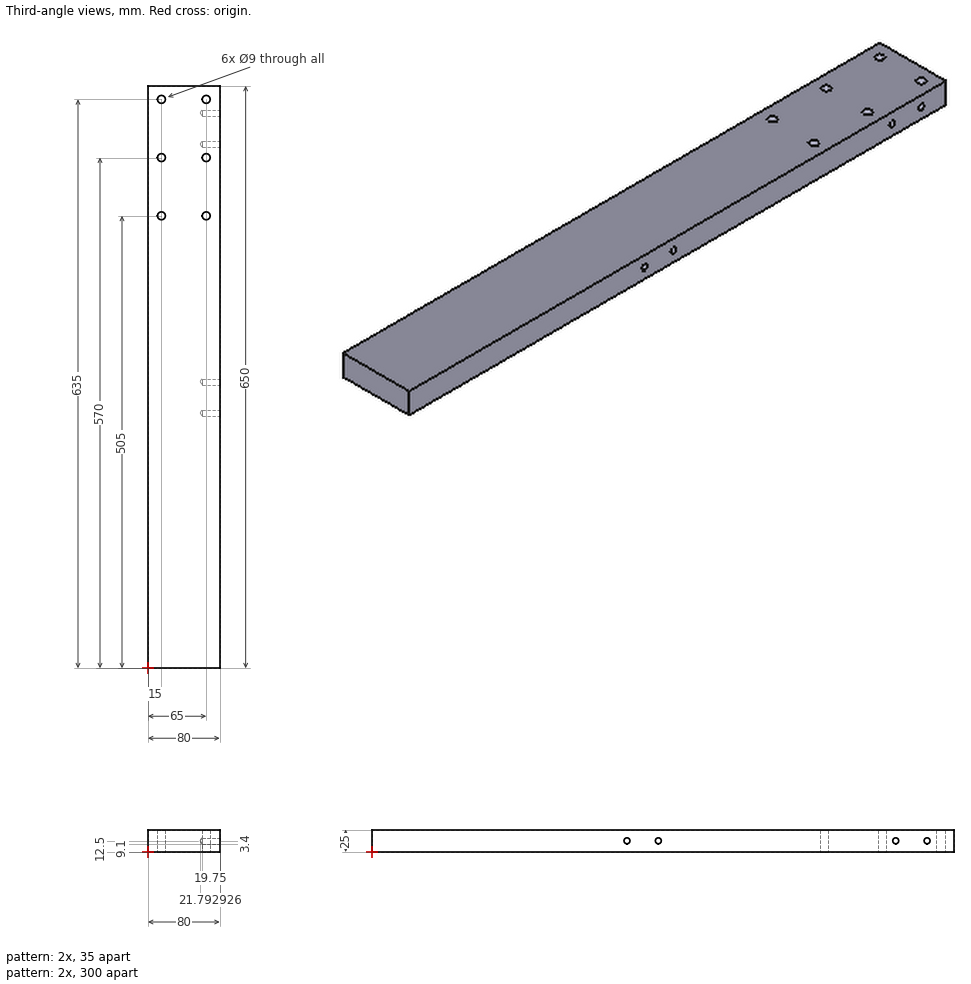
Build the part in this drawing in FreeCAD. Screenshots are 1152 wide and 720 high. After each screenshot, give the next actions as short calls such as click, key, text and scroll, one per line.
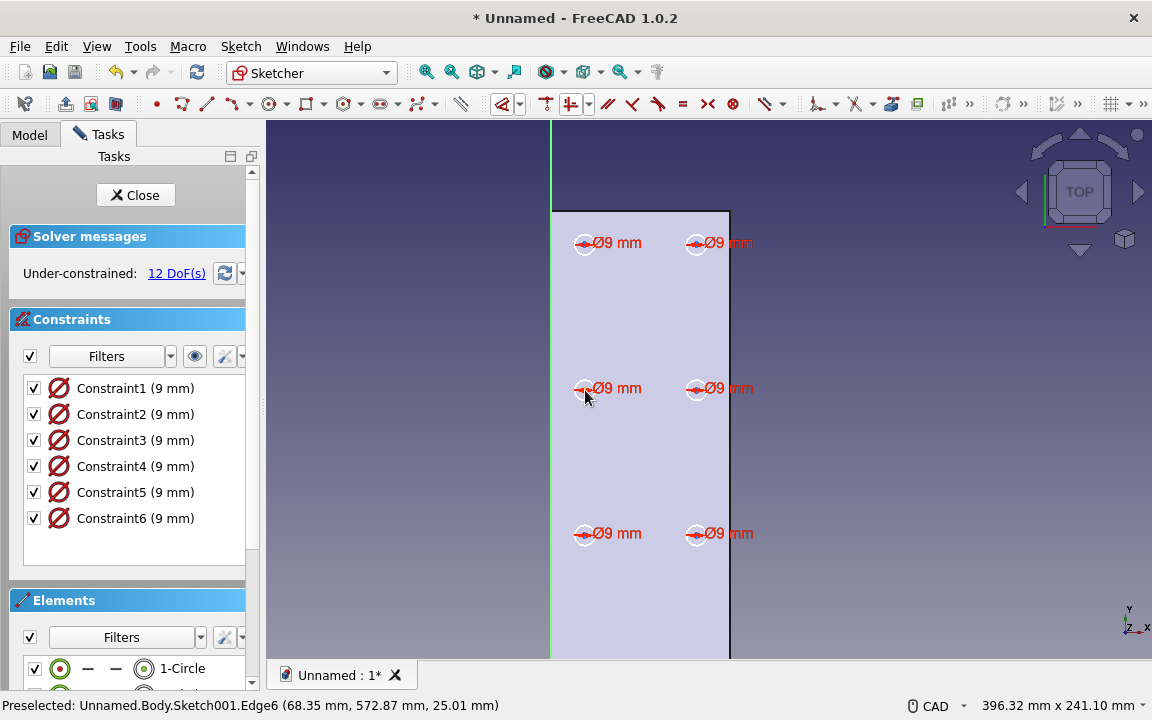
click(585, 245)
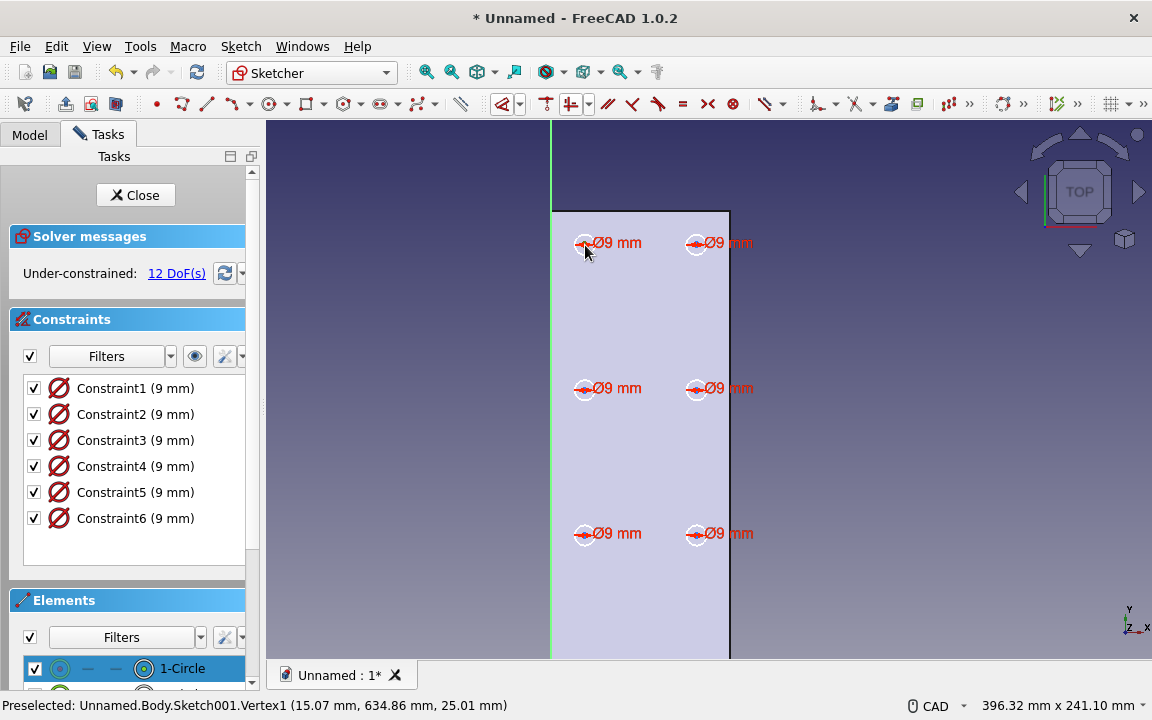
click(696, 245)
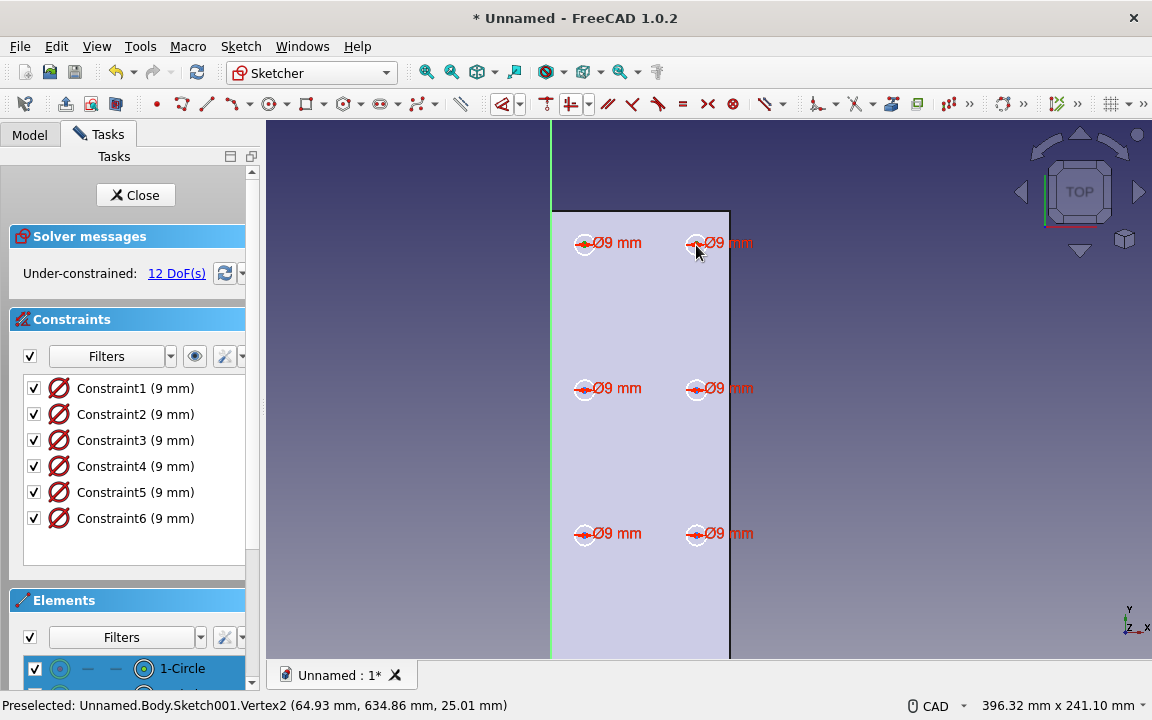
key(h)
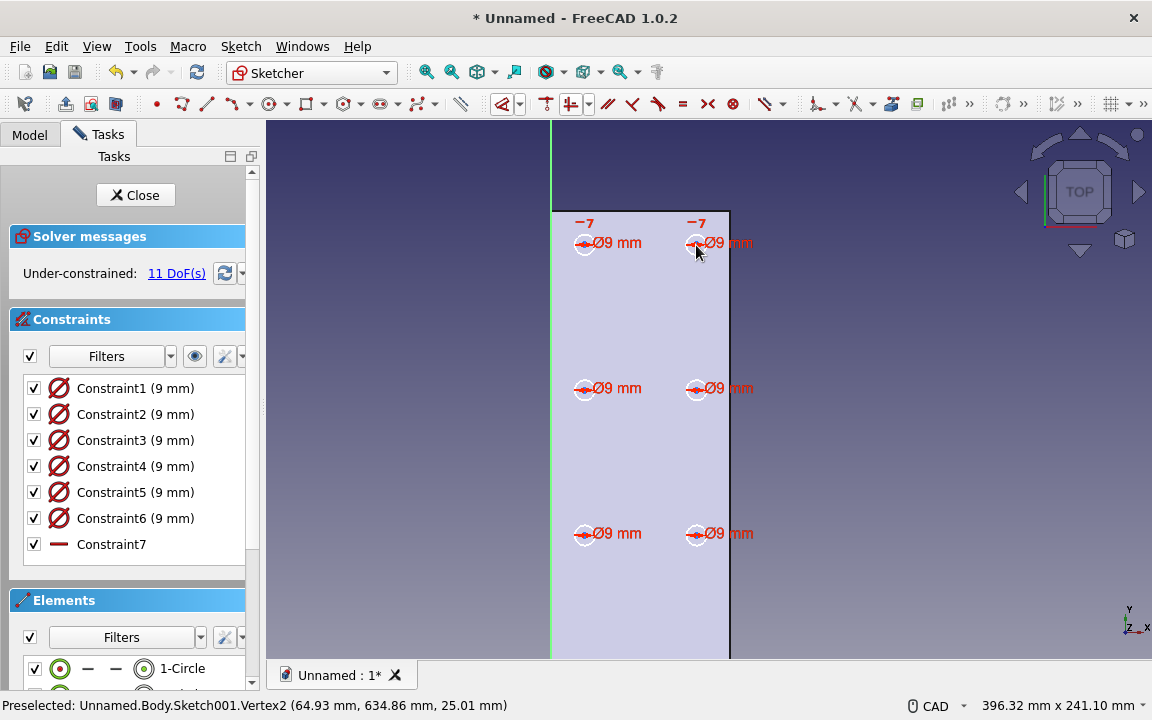
click(585, 245)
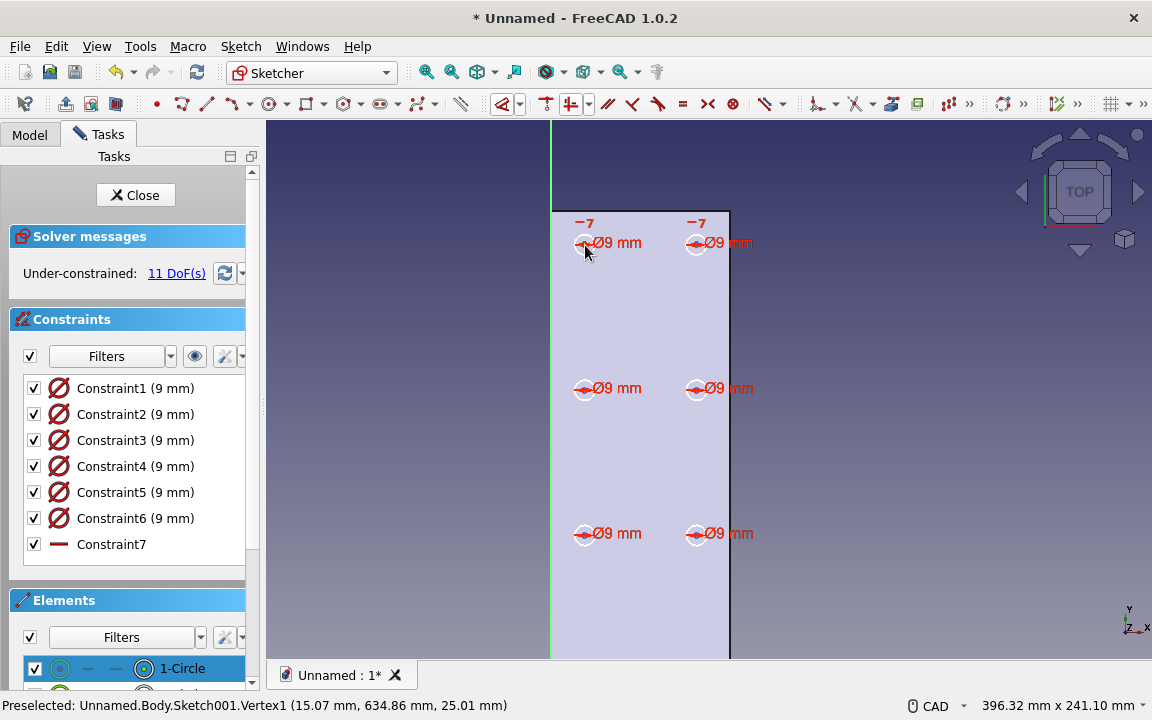
click(585, 535)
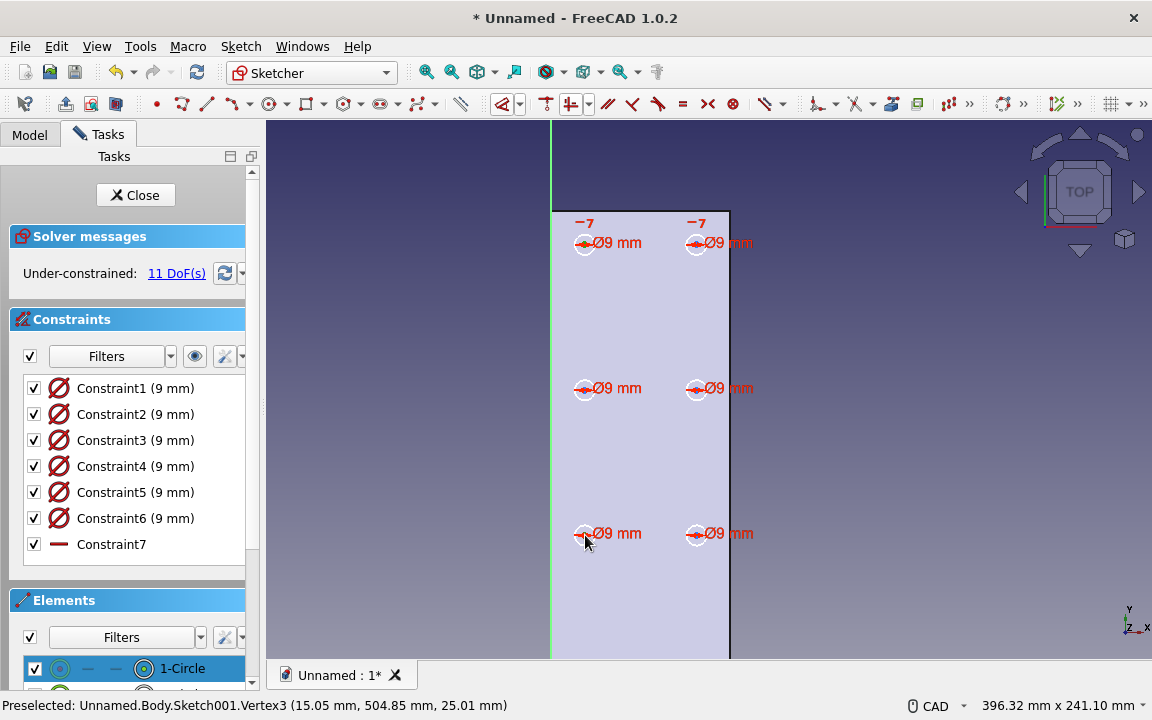
key(v)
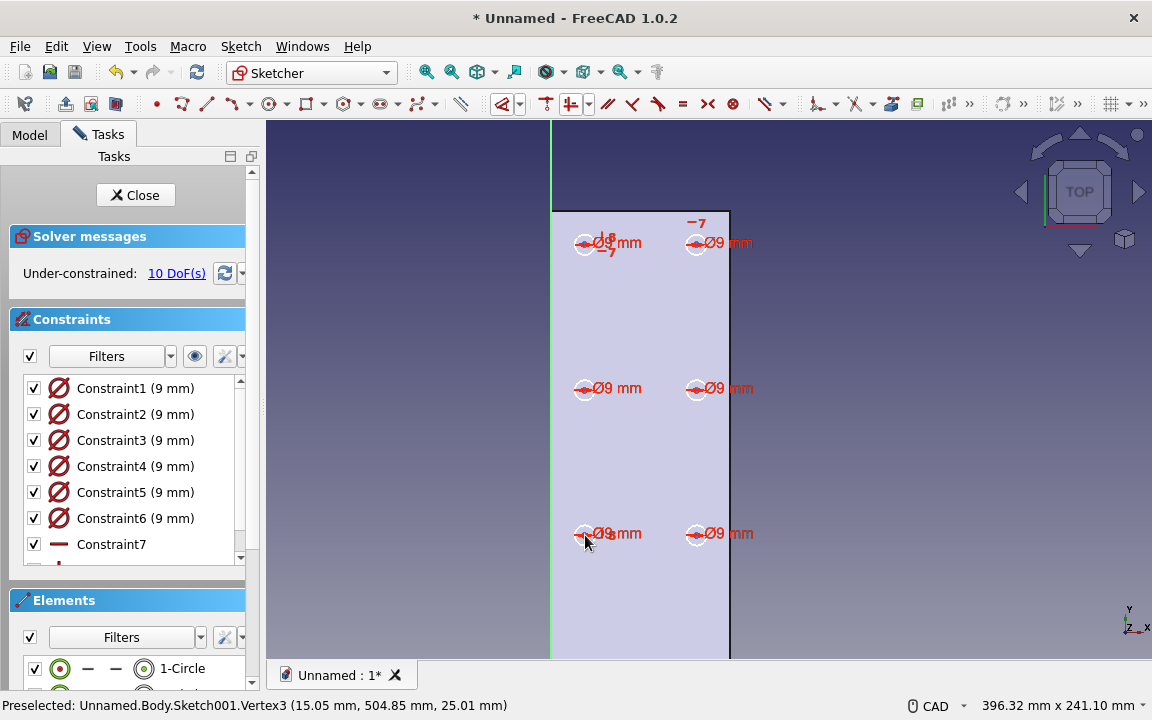
click(696, 245)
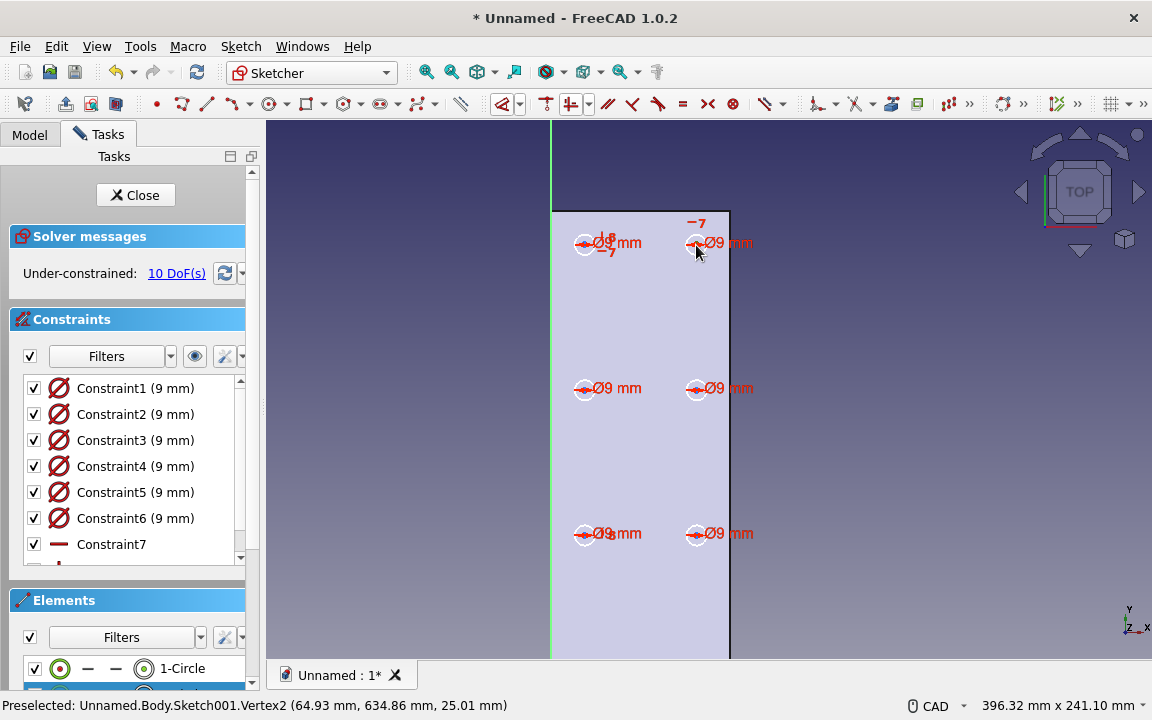
click(697, 535)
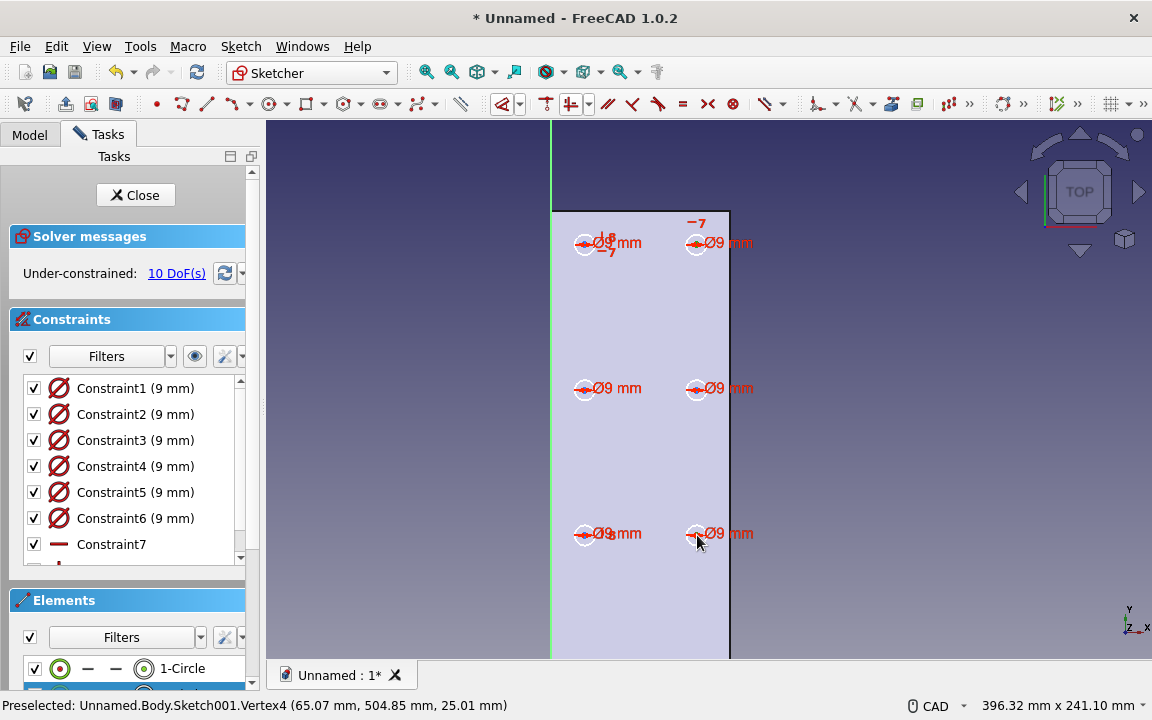
key(v)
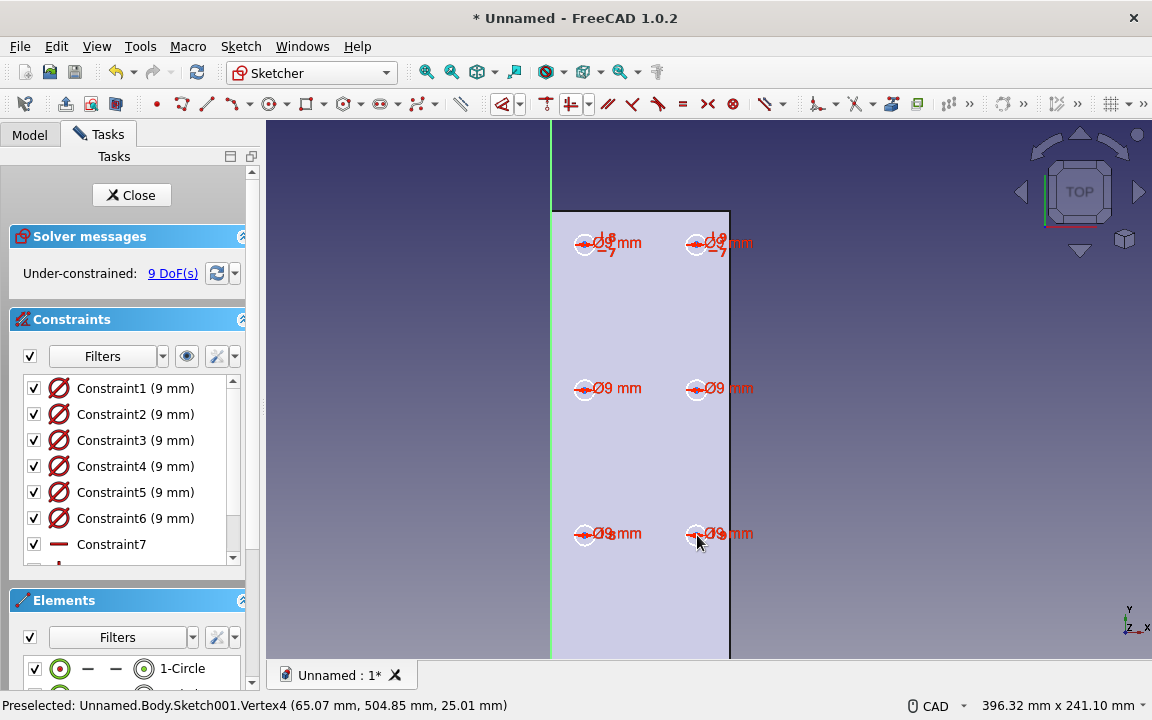
click(585, 535)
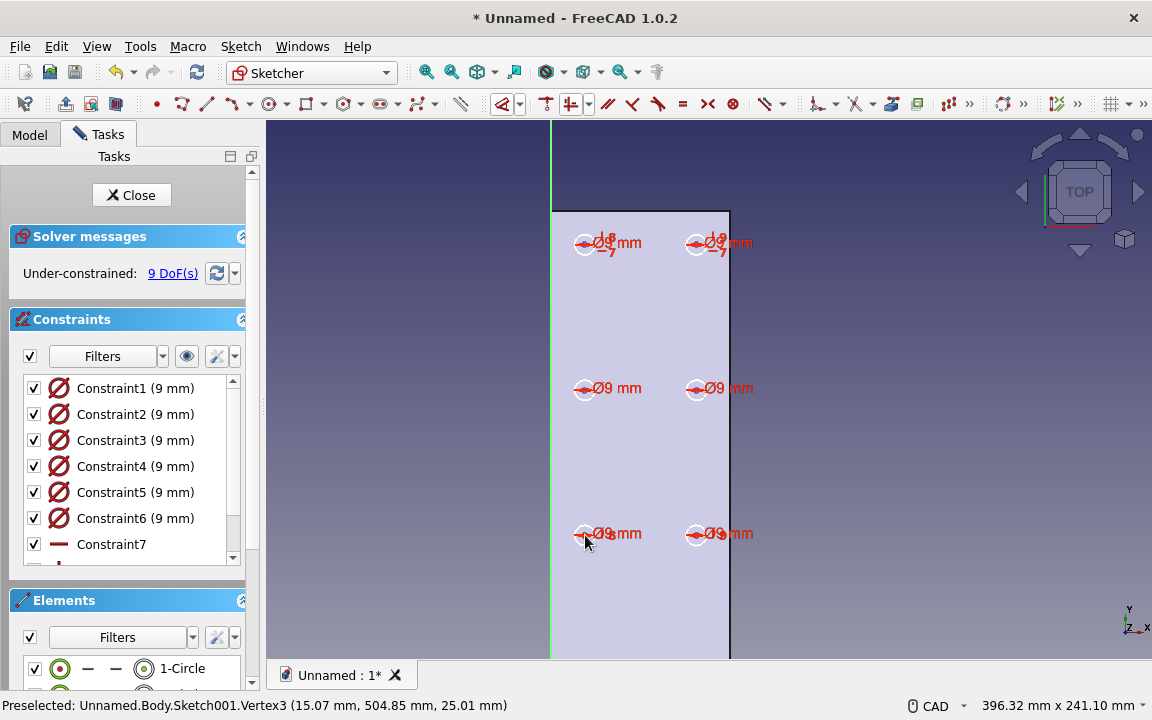
click(696, 535)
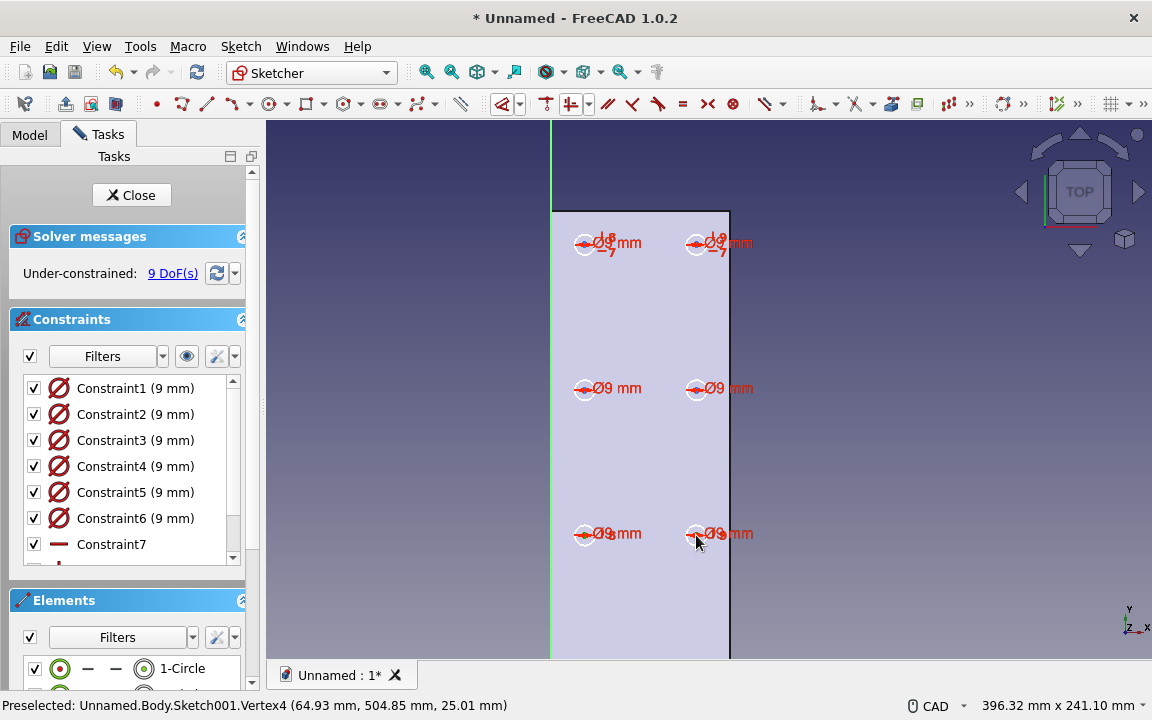
key(h)